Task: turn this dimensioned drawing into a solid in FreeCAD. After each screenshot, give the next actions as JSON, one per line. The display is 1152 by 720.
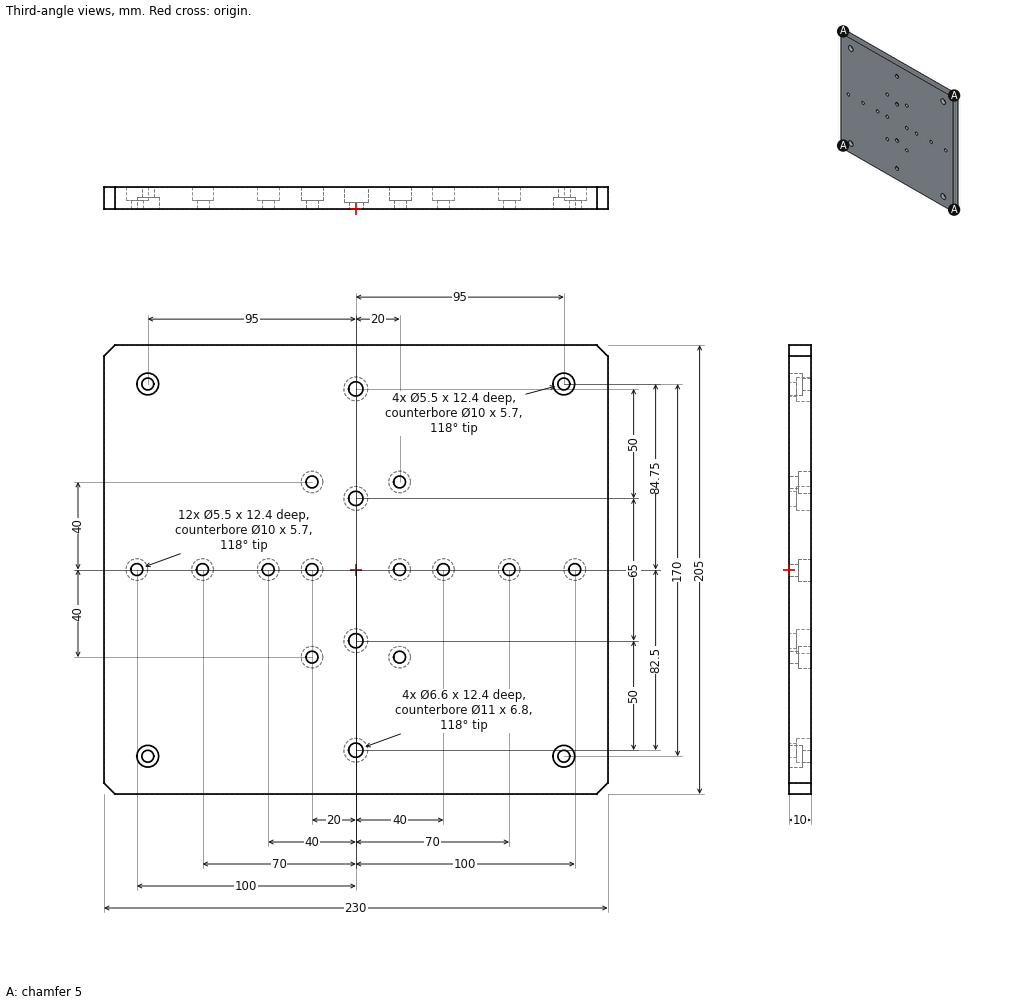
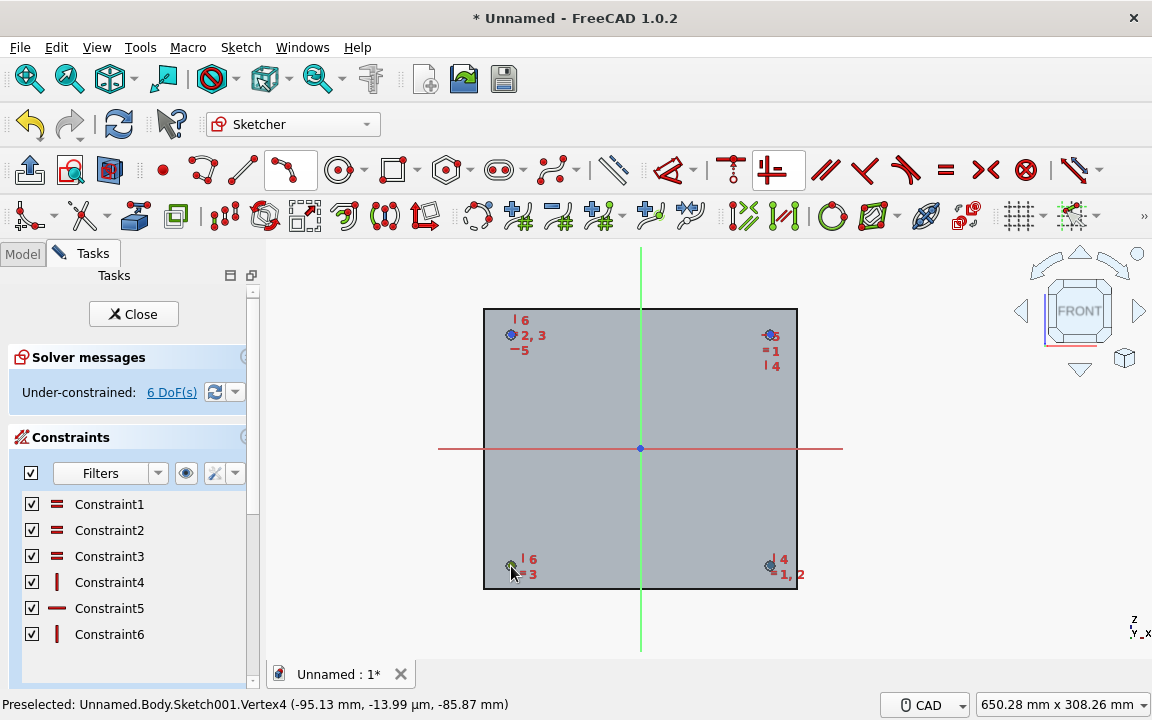
{"action": "key", "text": "h"}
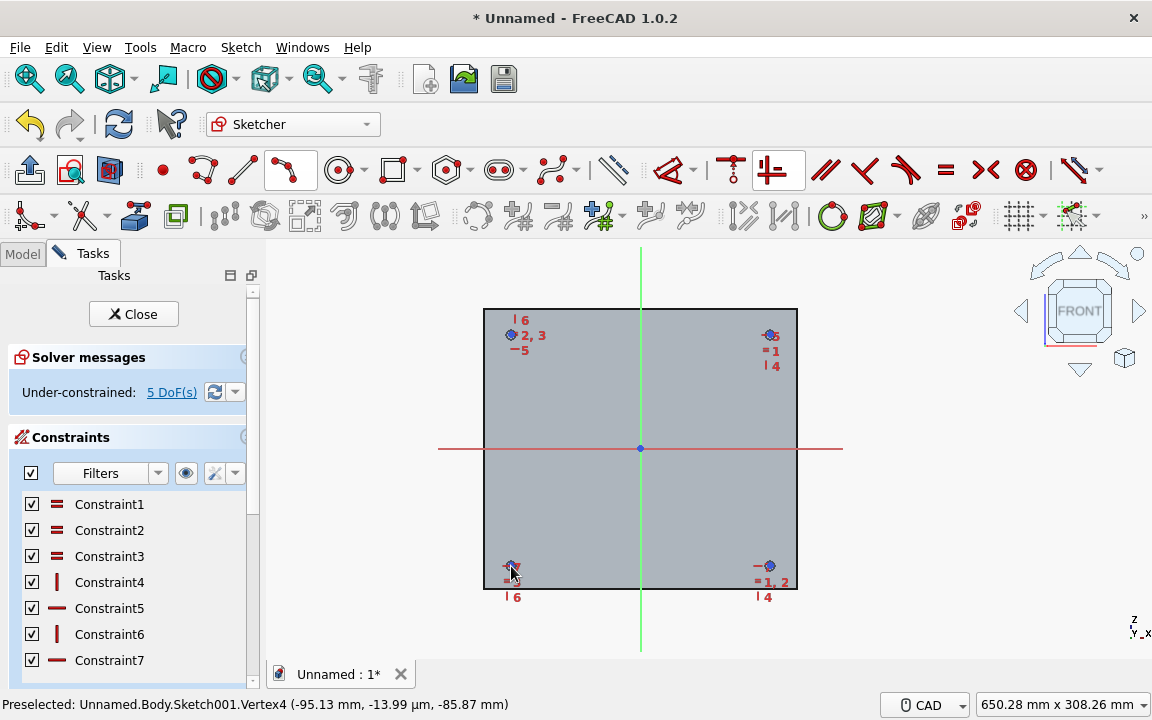
{"action": "left_click", "coordinate": [668, 170]}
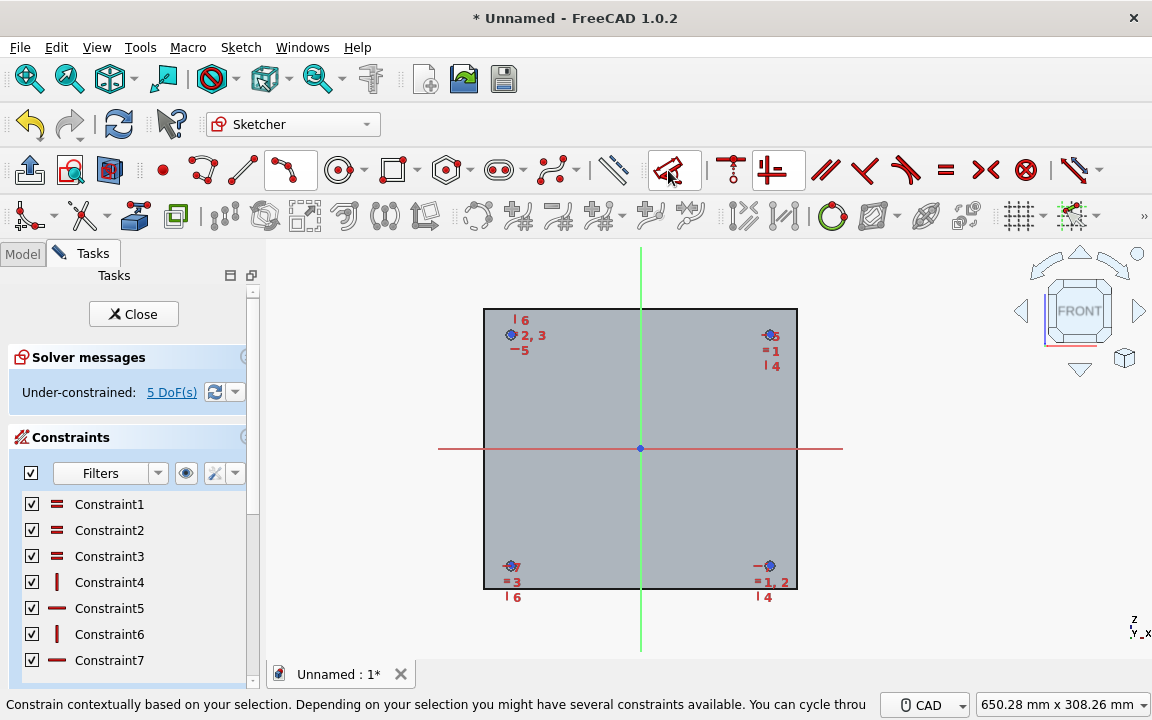
{"action": "scroll", "coordinate": [767, 332], "scroll_direction": "up", "scroll_amount": 9}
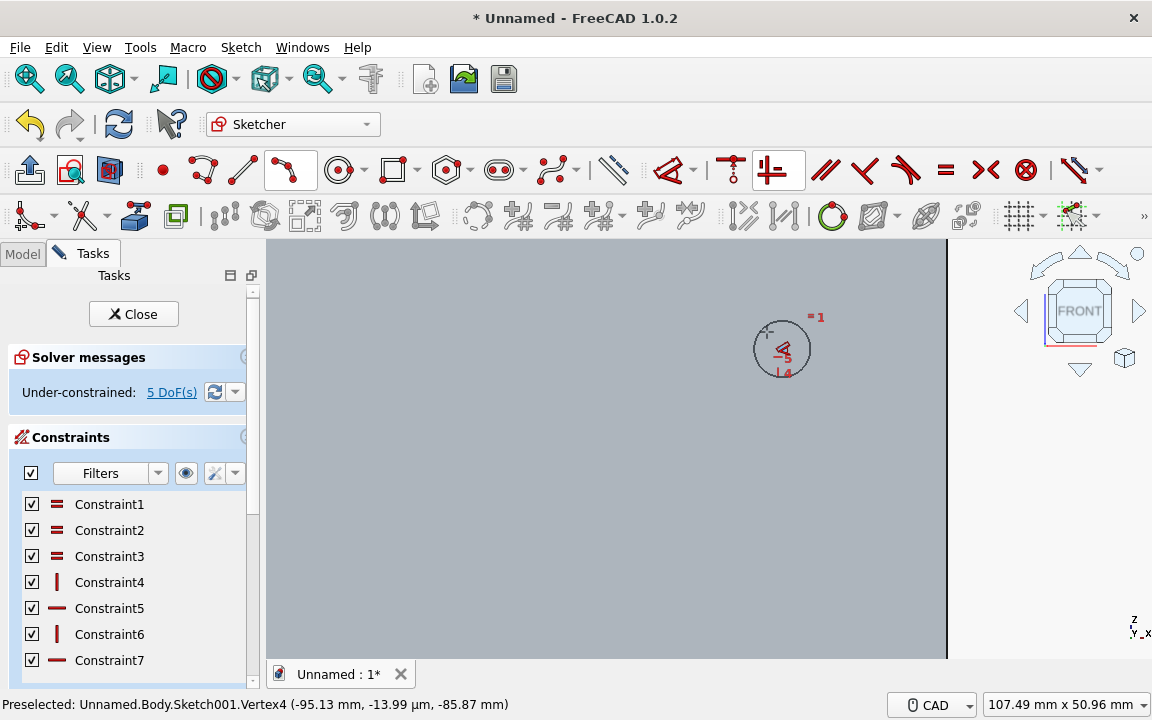
{"action": "left_click", "coordinate": [762, 329]}
{"action": "left_click", "coordinate": [739, 307]}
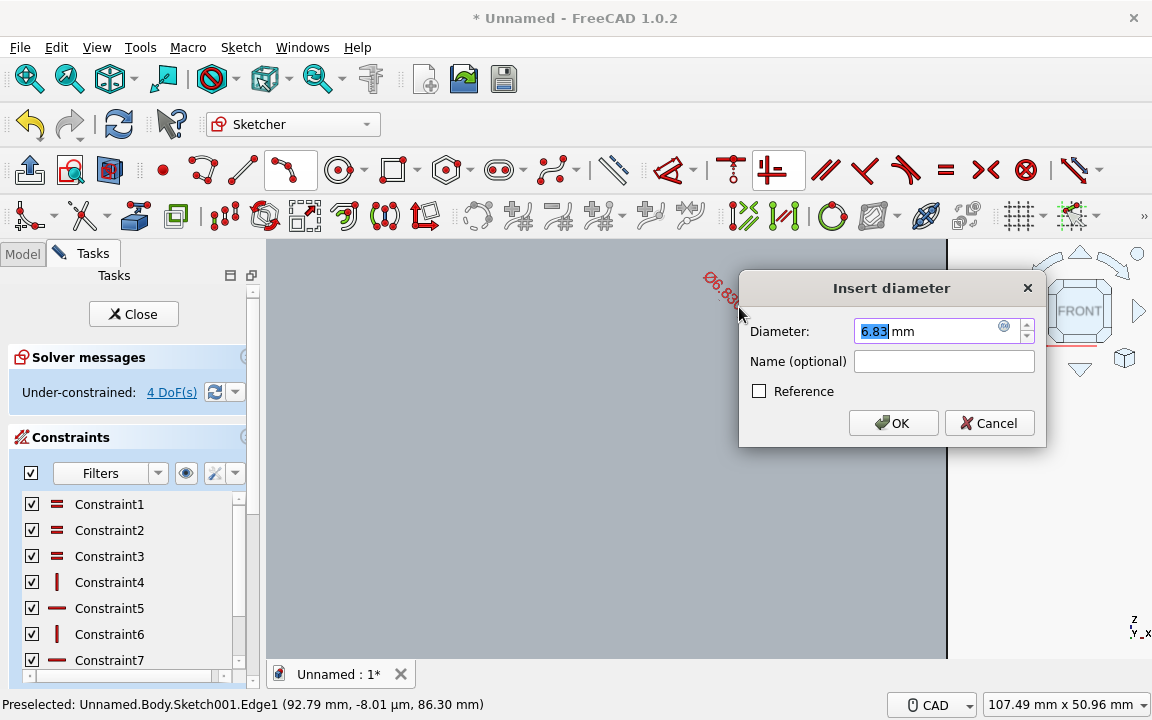
{"action": "type", "text": "5.5"}
{"action": "key", "text": "Return"}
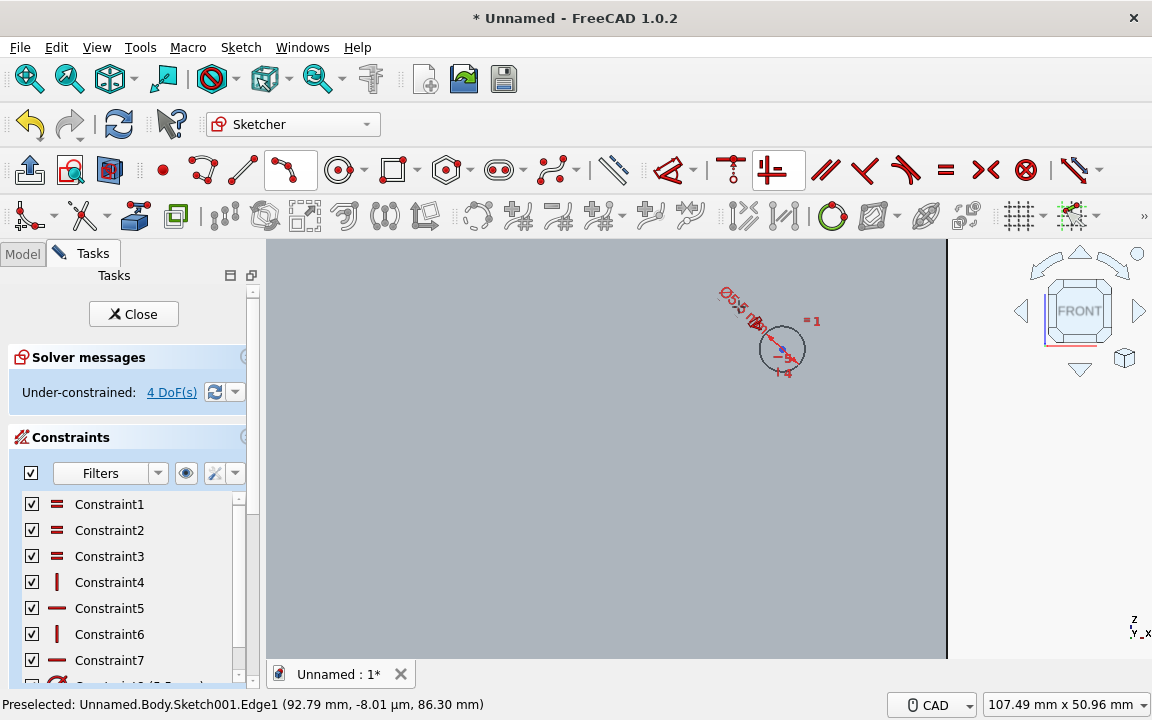
{"action": "scroll", "coordinate": [767, 332], "scroll_direction": "down", "scroll_amount": 9}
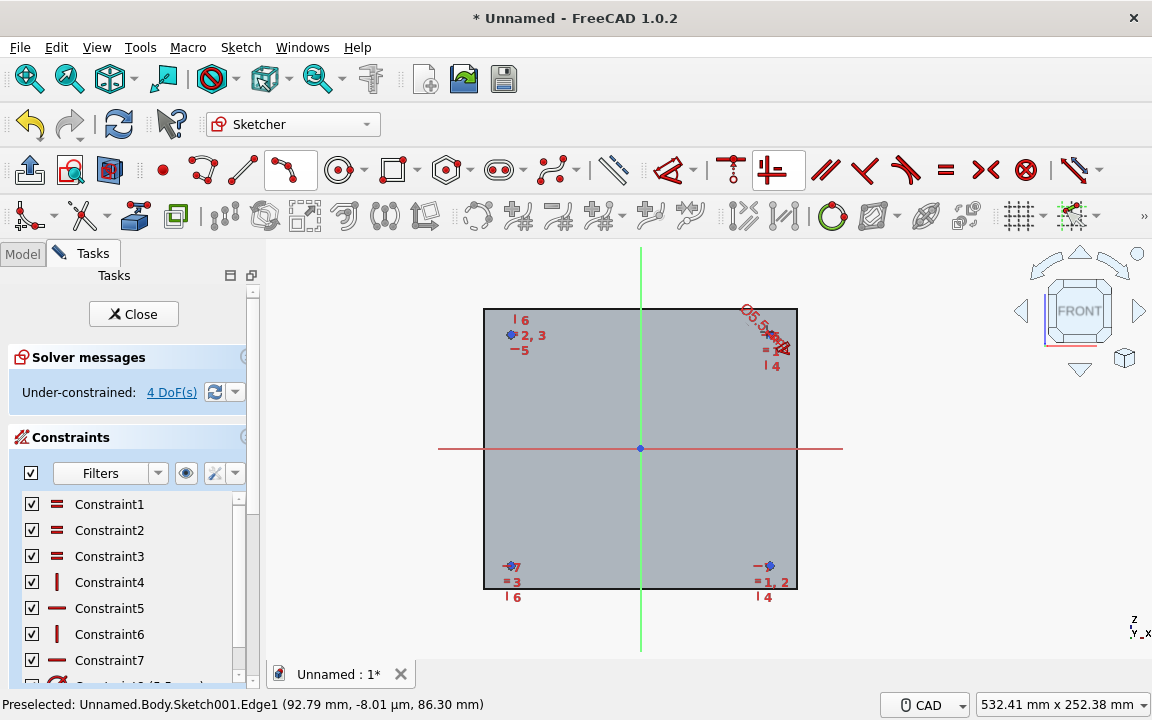
{"action": "left_click", "coordinate": [770, 335]}
{"action": "left_click", "coordinate": [705, 301]}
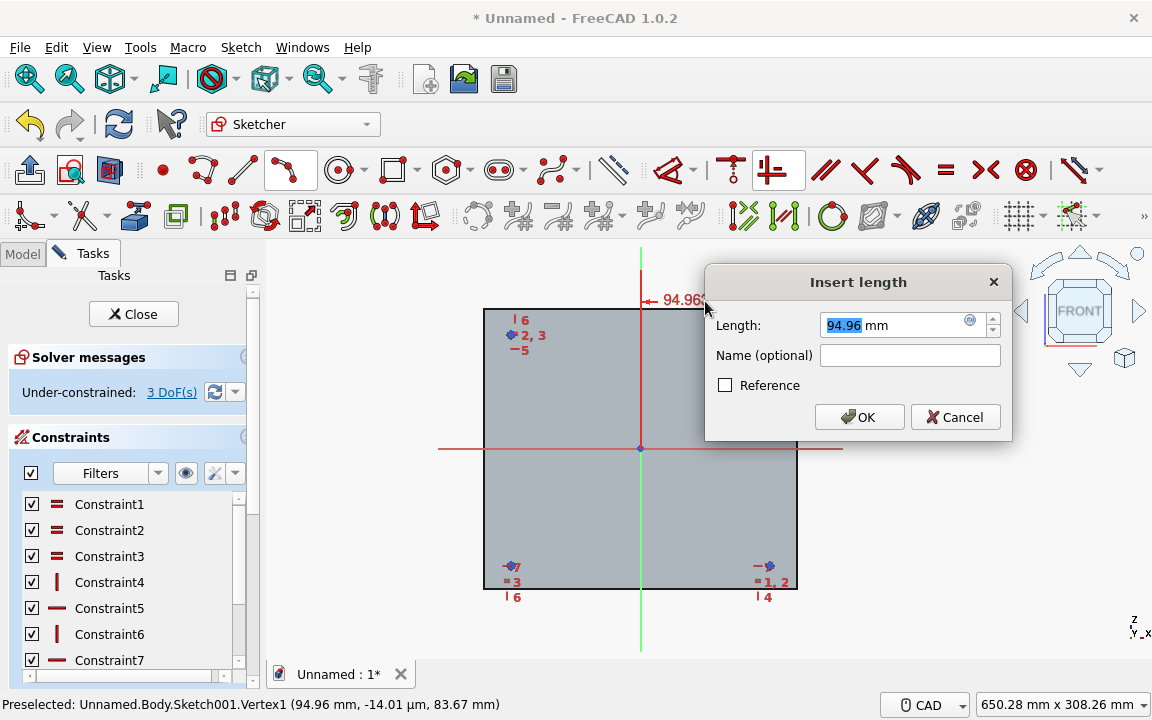
{"action": "type", "text": "95"}
{"action": "key", "text": "Return"}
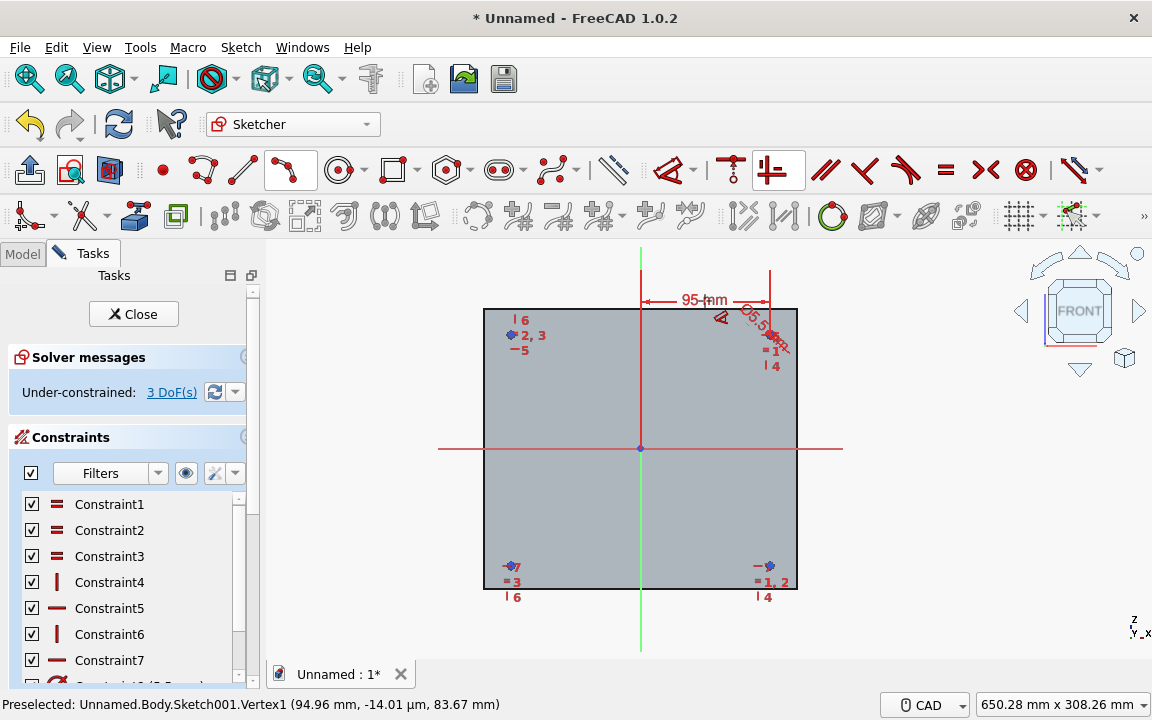
{"action": "left_click", "coordinate": [511, 335]}
{"action": "left_click", "coordinate": [576, 301]}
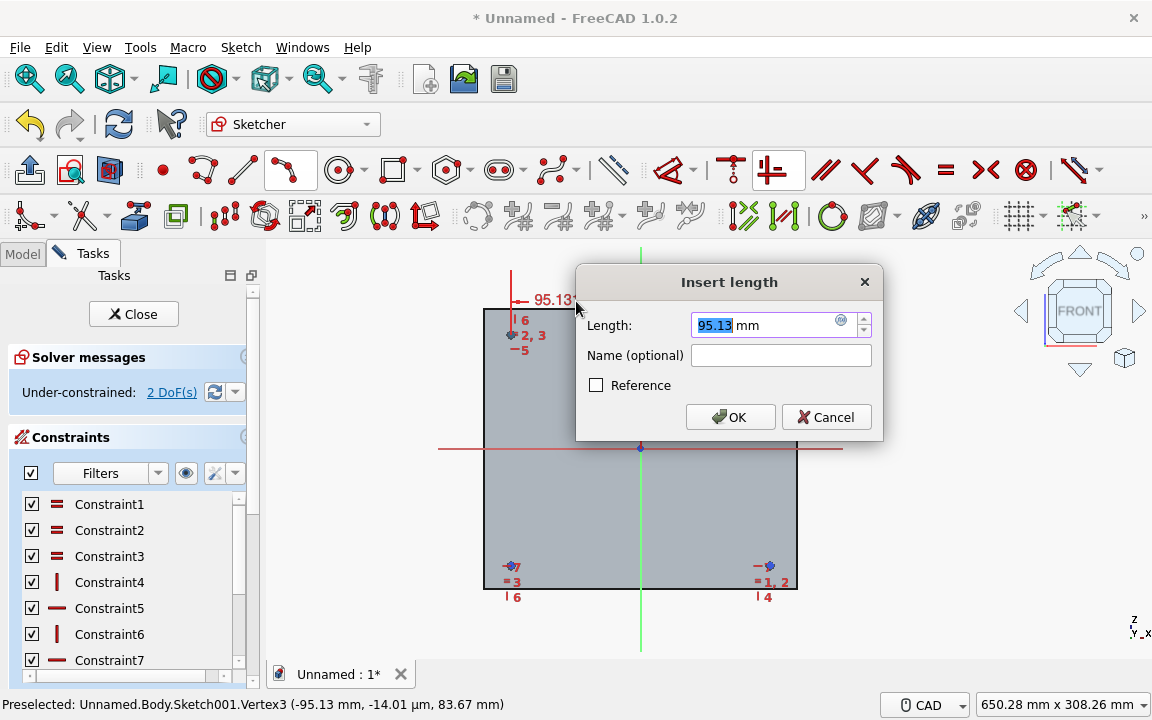
{"action": "type", "text": "95"}
{"action": "key", "text": "Return"}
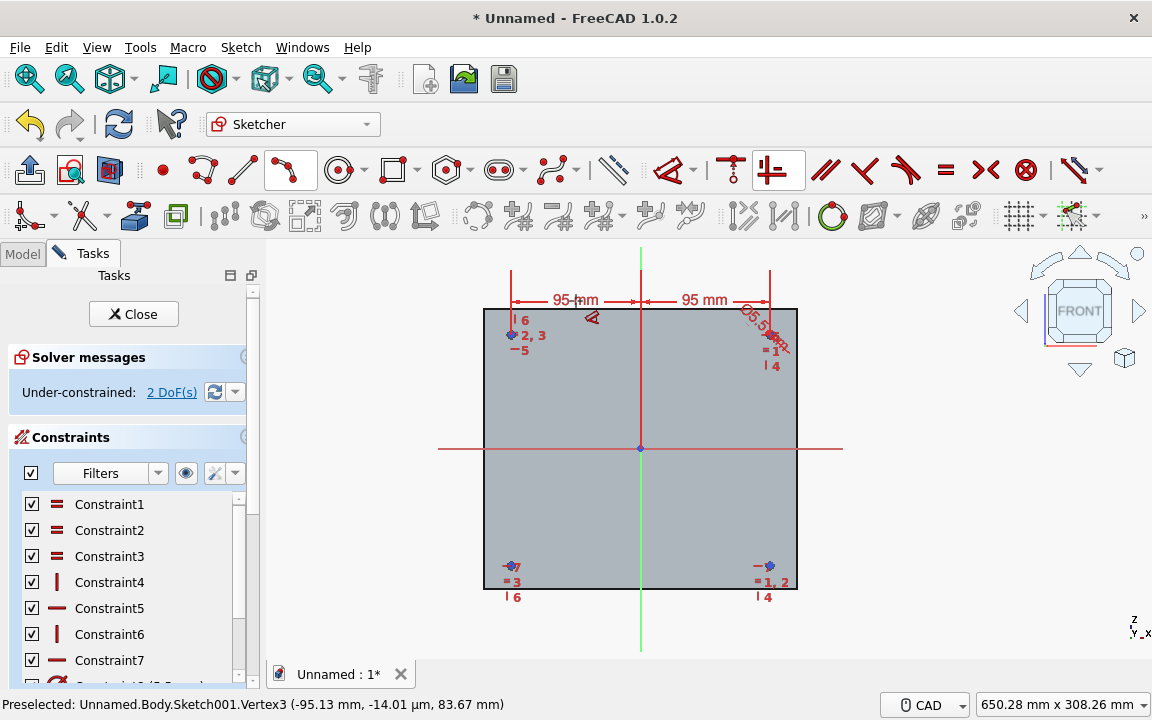
{"action": "left_click", "coordinate": [770, 335]}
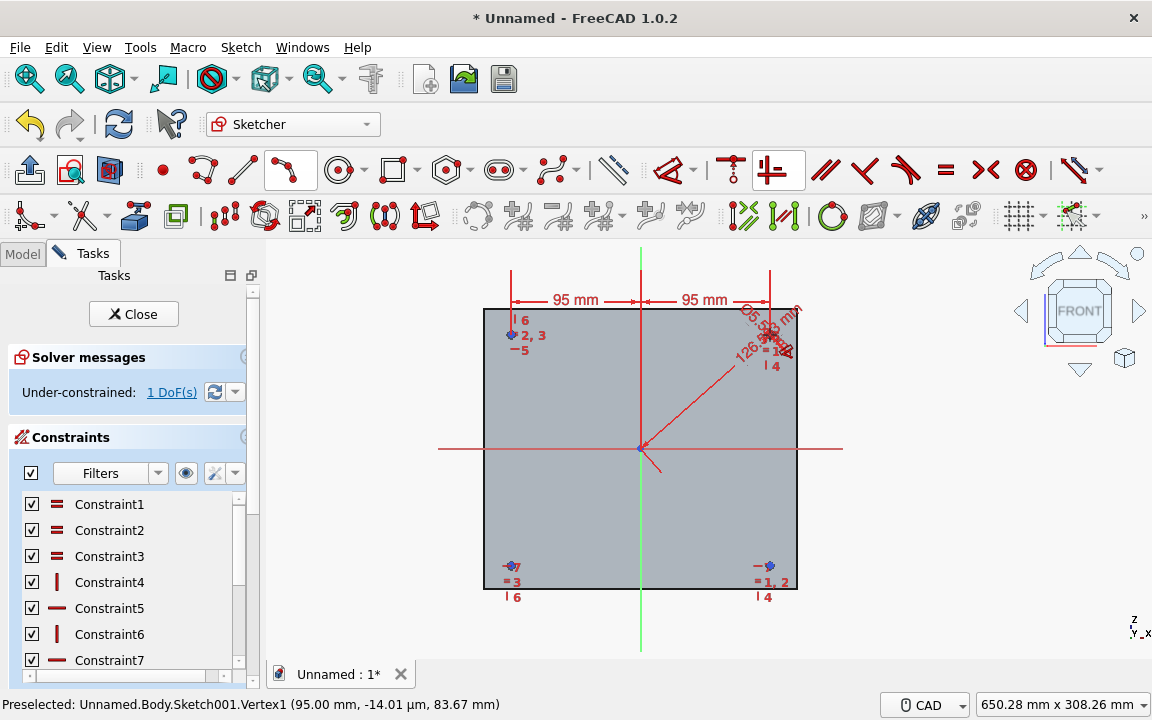
{"action": "left_click", "coordinate": [770, 566]}
{"action": "left_click", "coordinate": [804, 397]}